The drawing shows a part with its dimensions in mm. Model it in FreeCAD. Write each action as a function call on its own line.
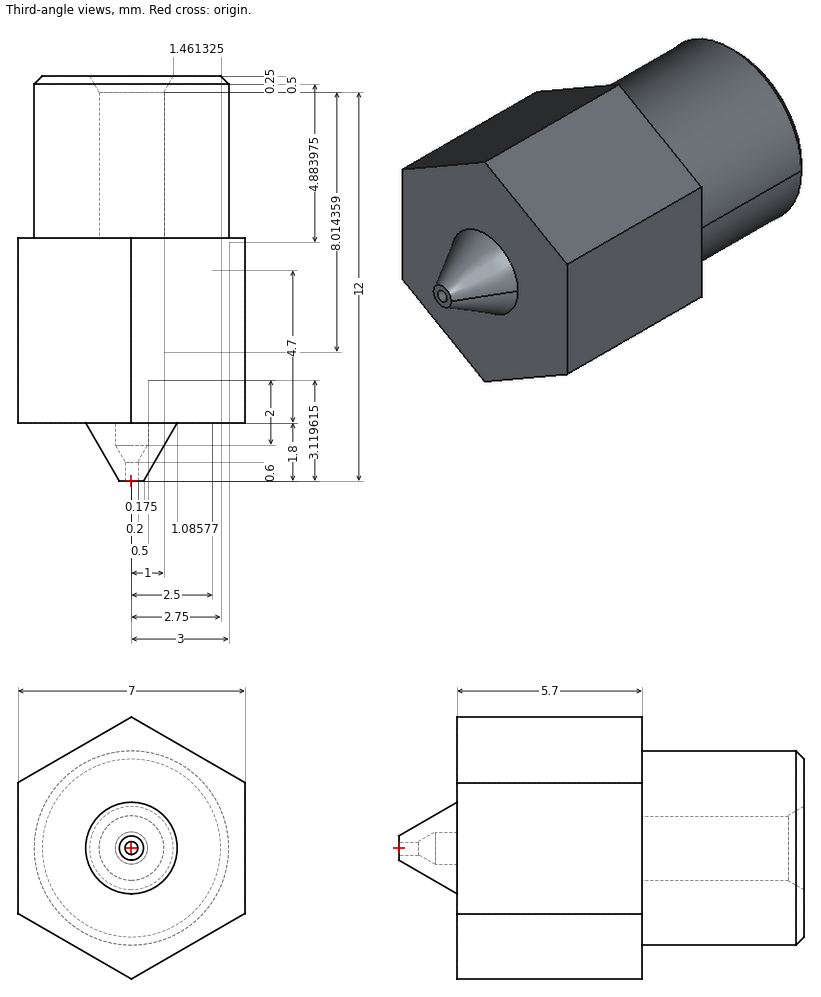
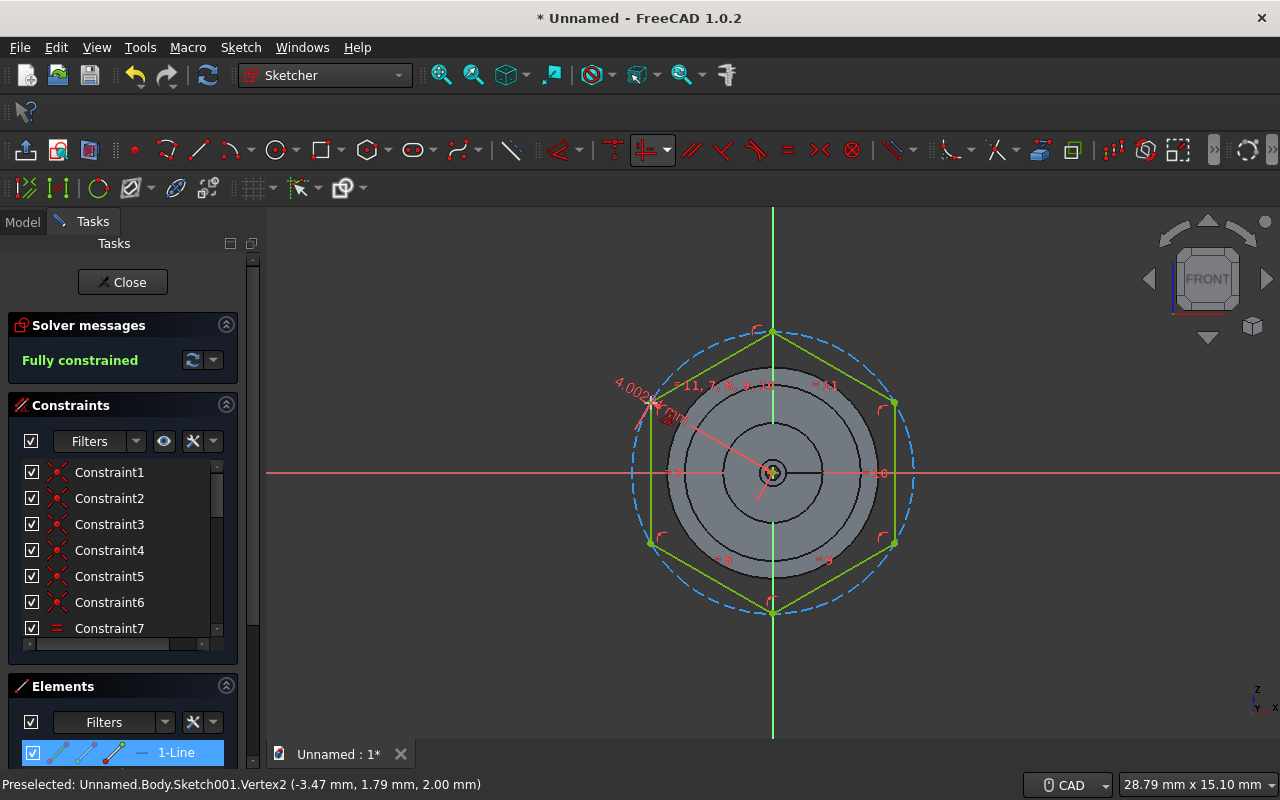
click(895, 544)
click(687, 602)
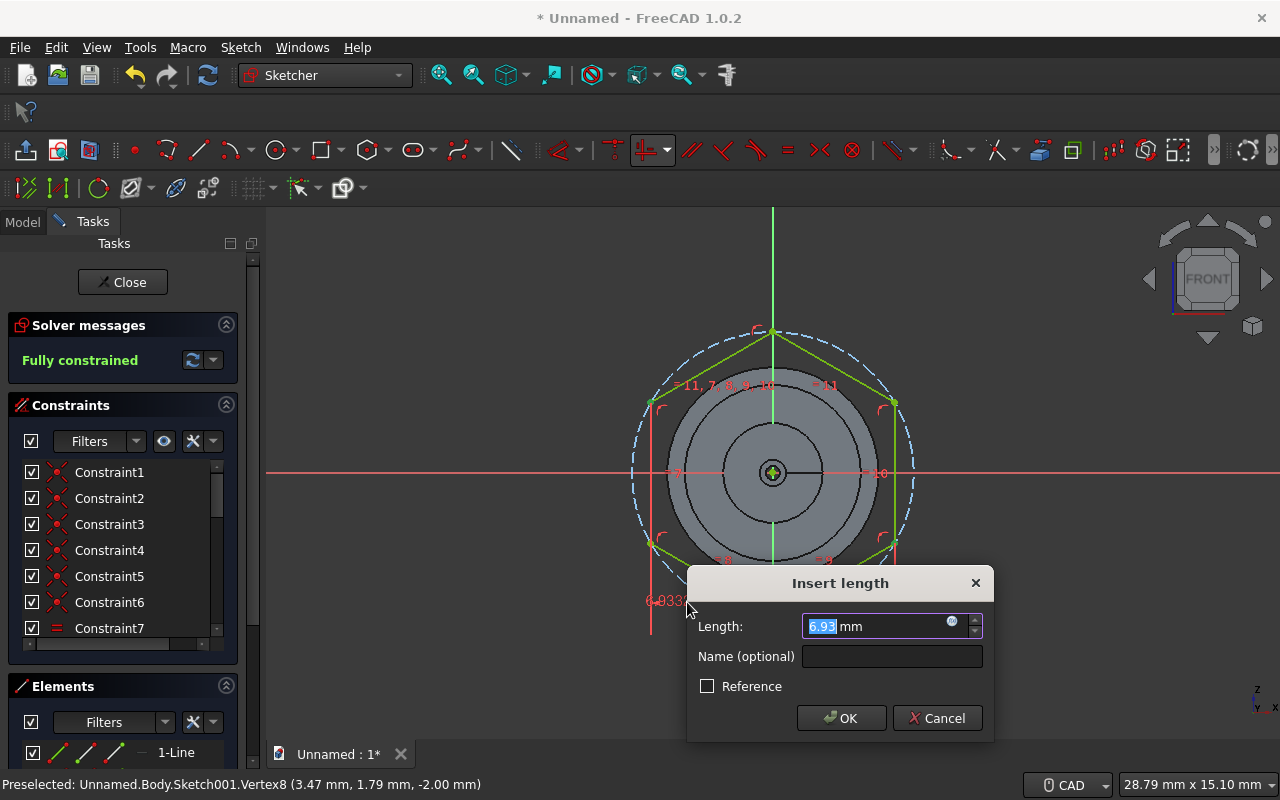
text(7)
key(Return)
key(Escape)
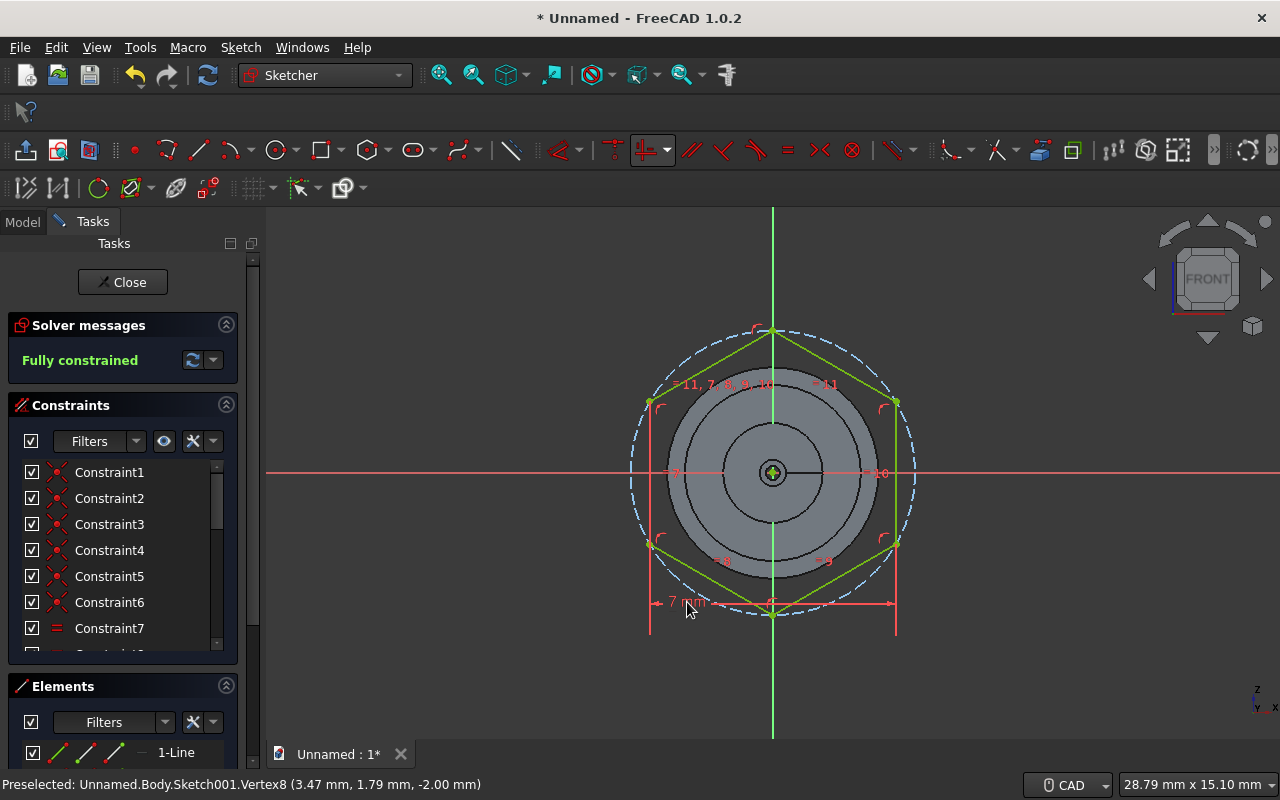
click(123, 282)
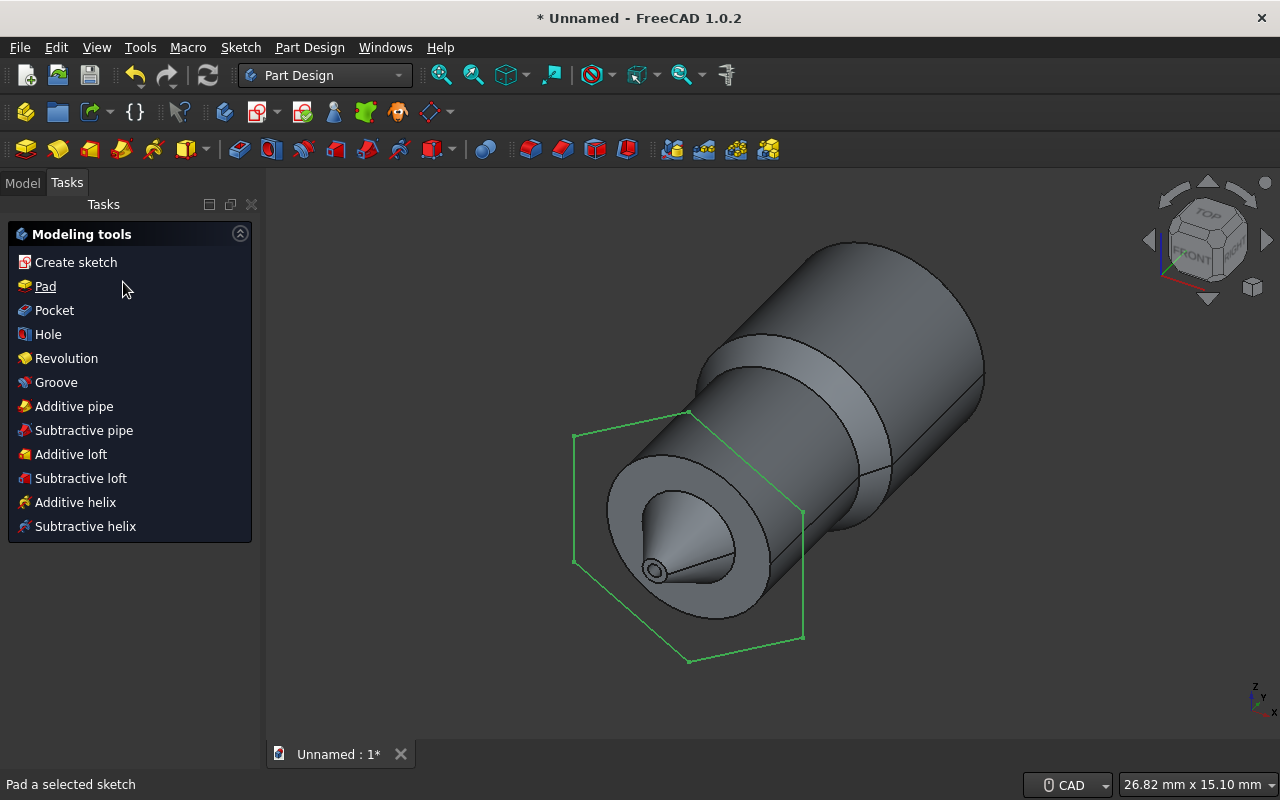
click(26, 150)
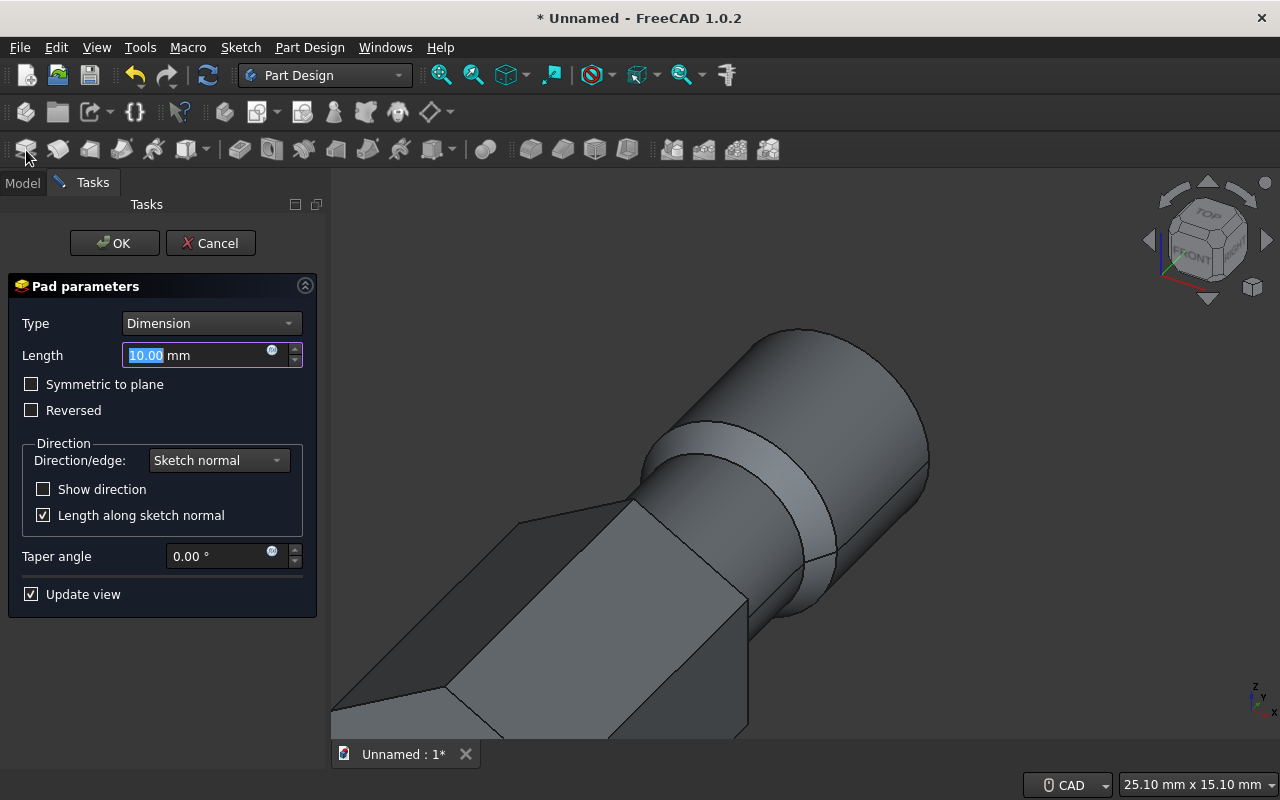
text(5.7)
key(Tab)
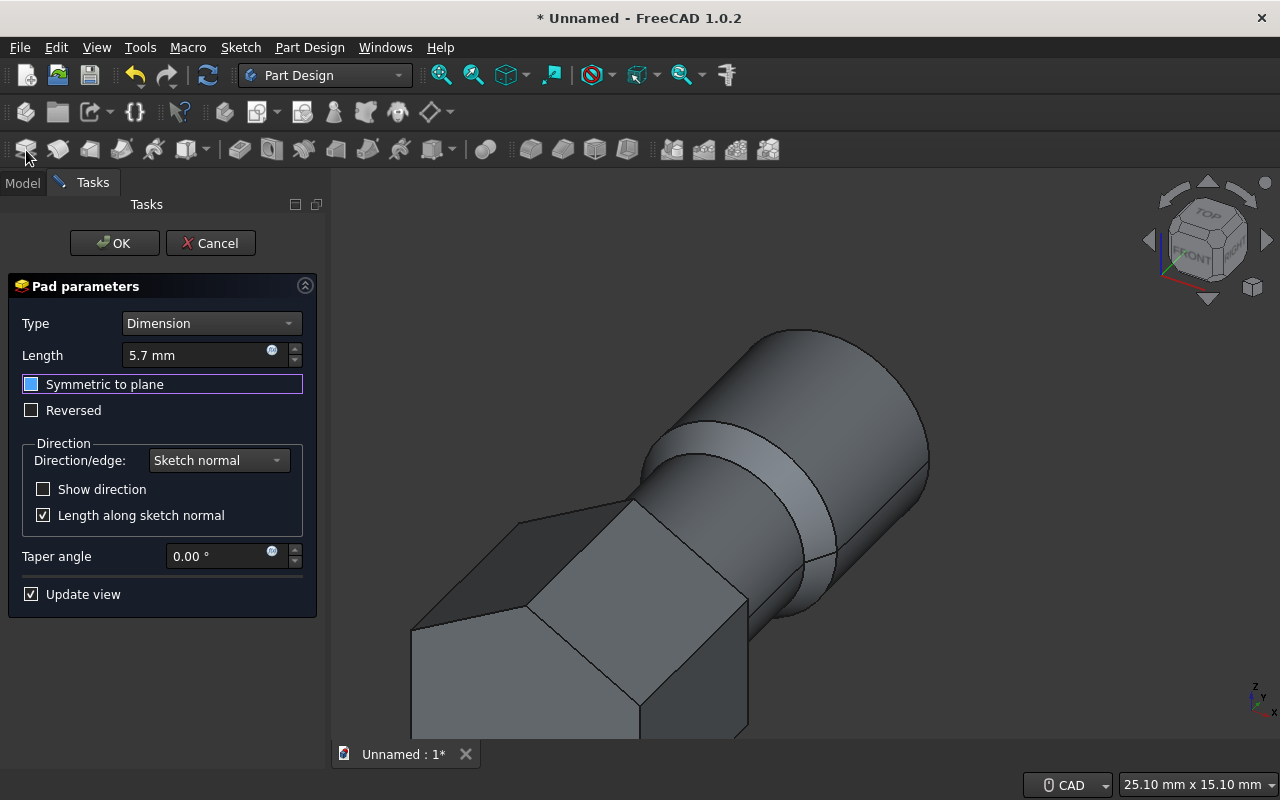
click(30, 410)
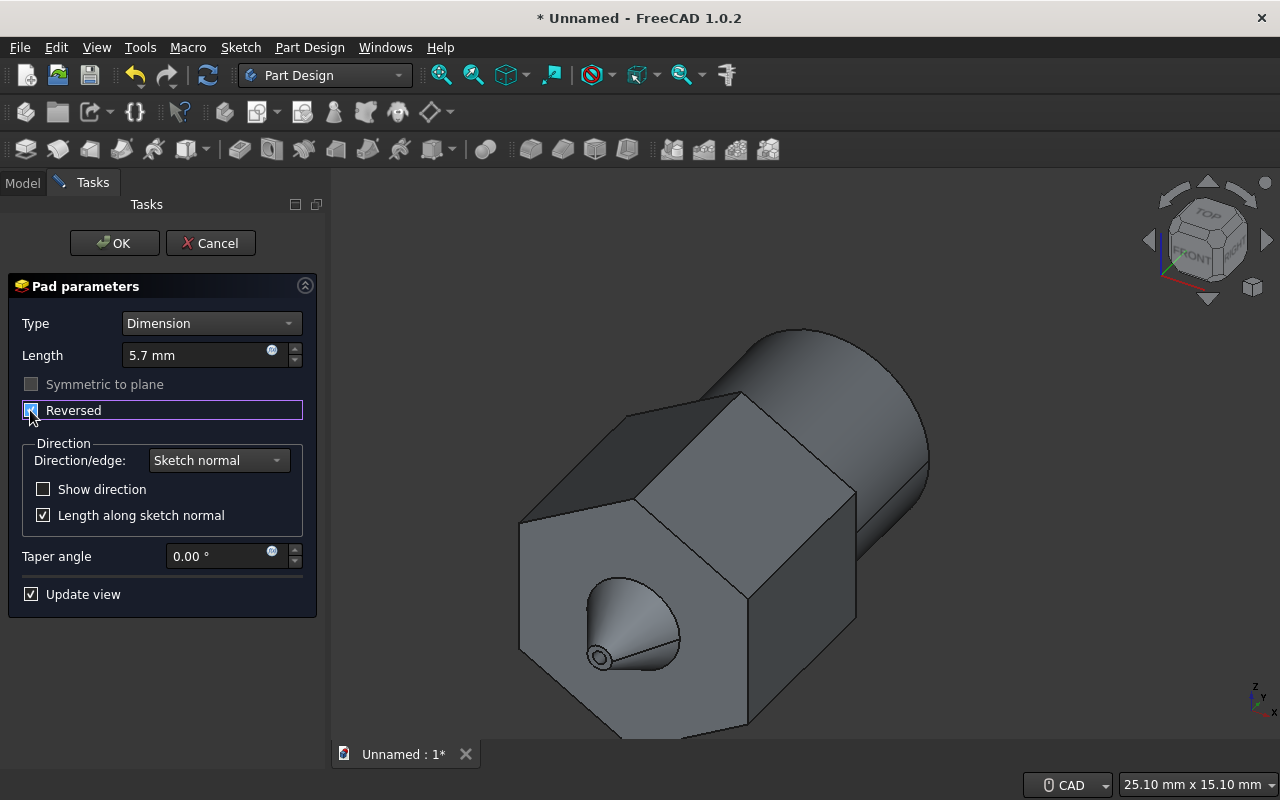
click(115, 243)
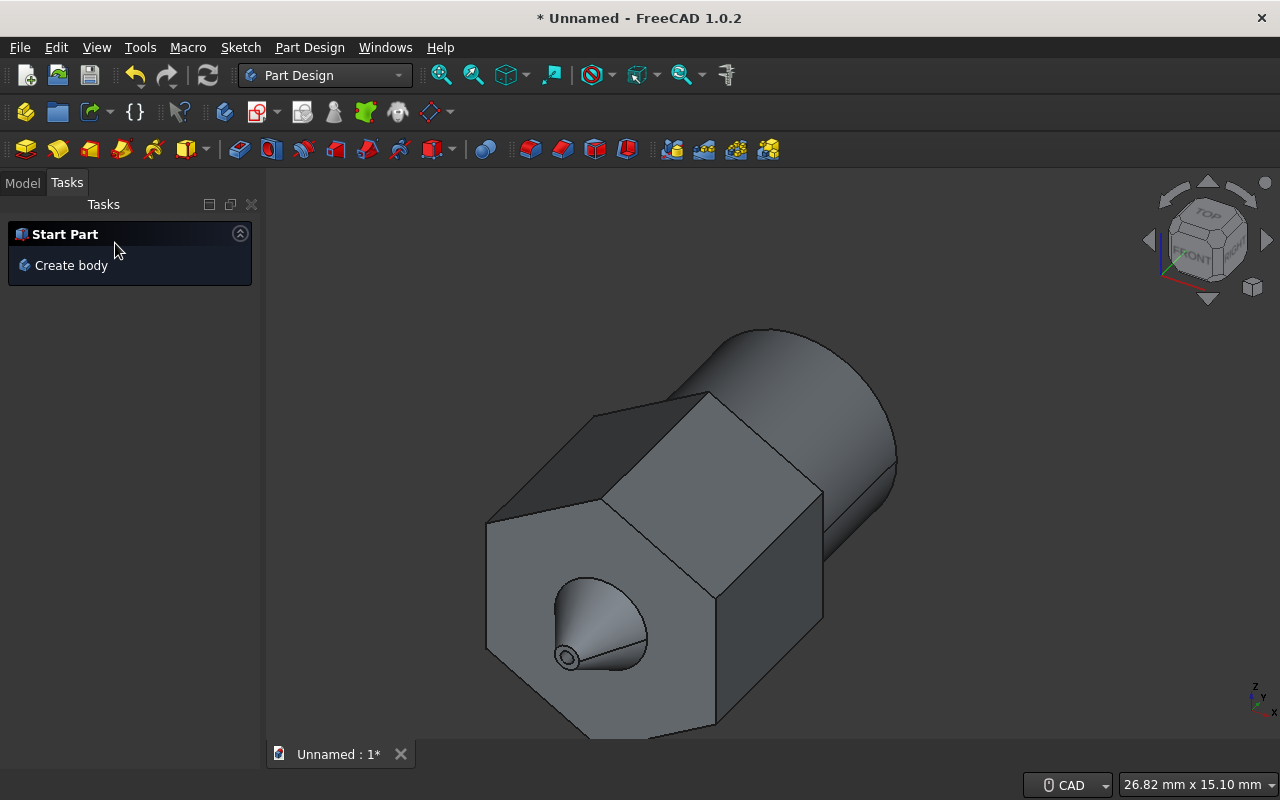
key(0)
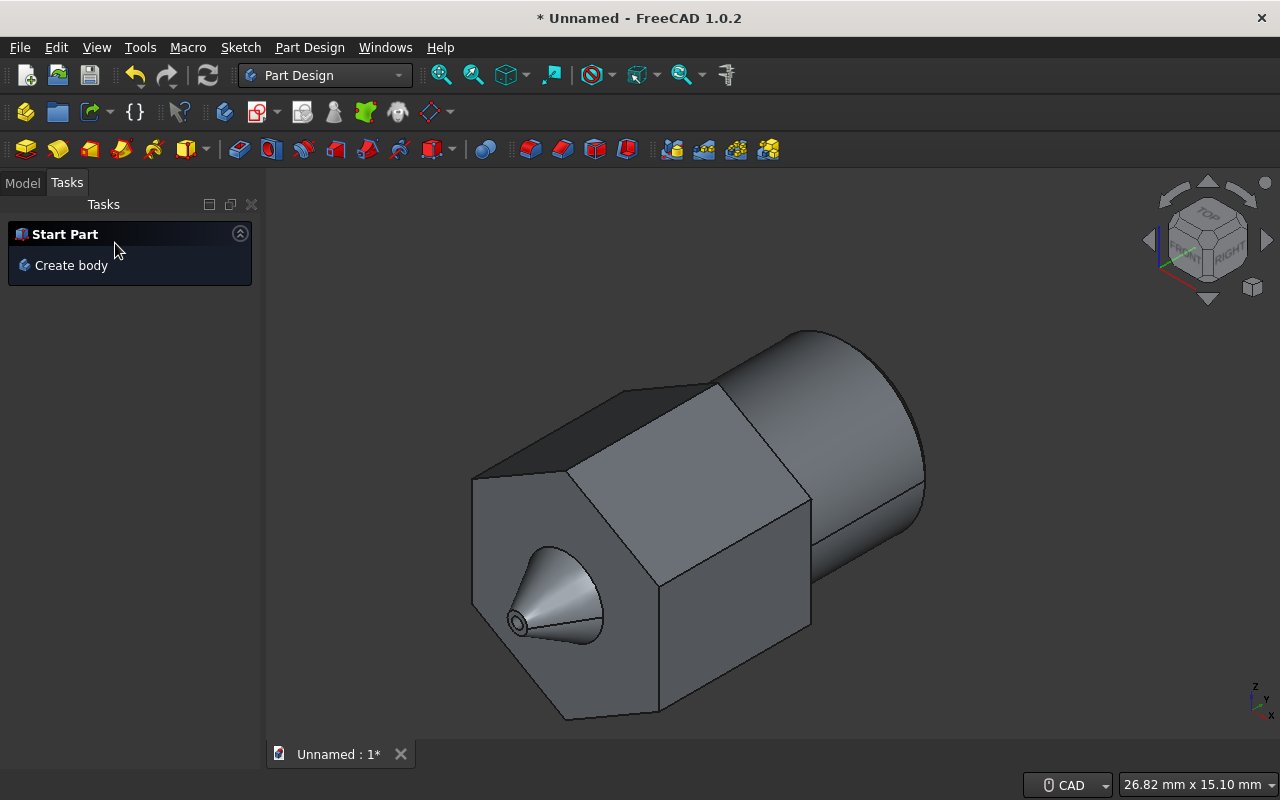
click(442, 76)